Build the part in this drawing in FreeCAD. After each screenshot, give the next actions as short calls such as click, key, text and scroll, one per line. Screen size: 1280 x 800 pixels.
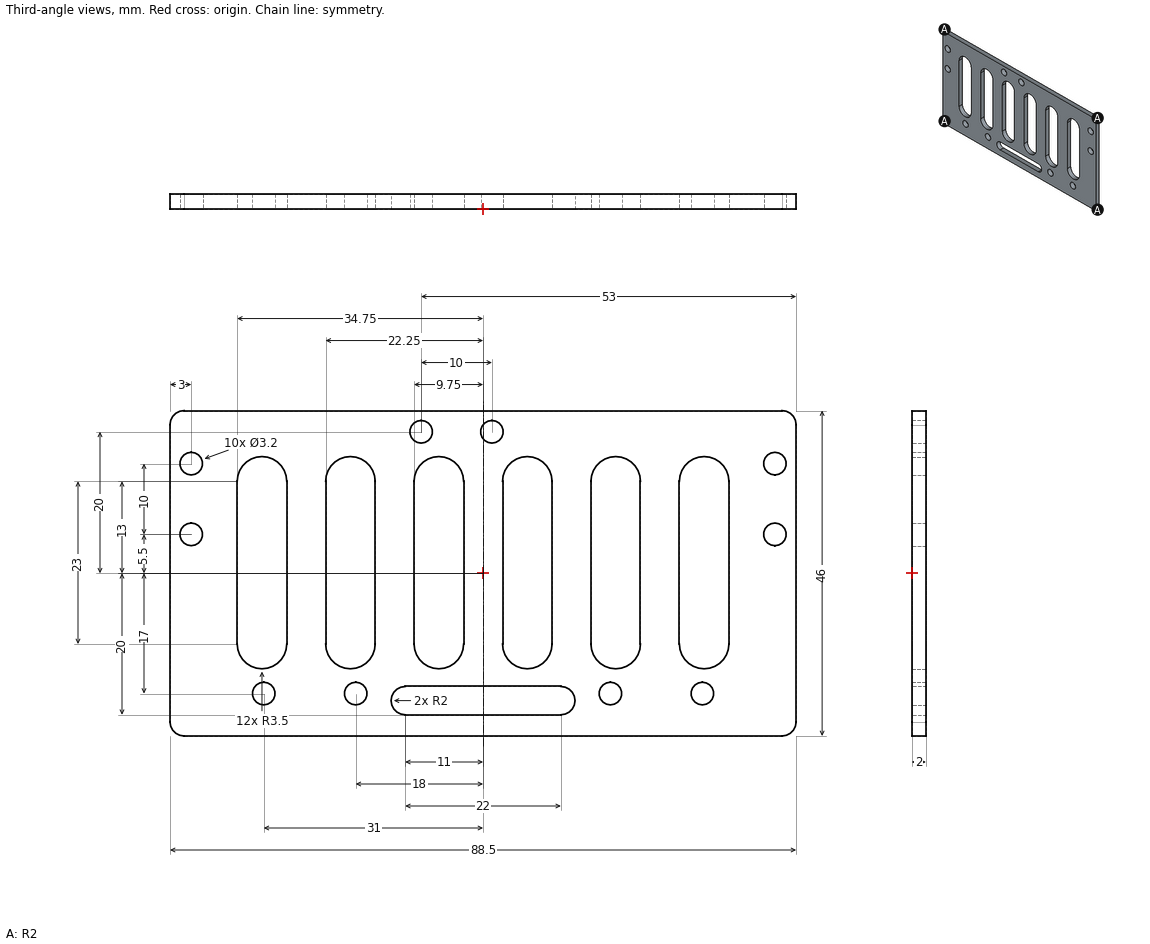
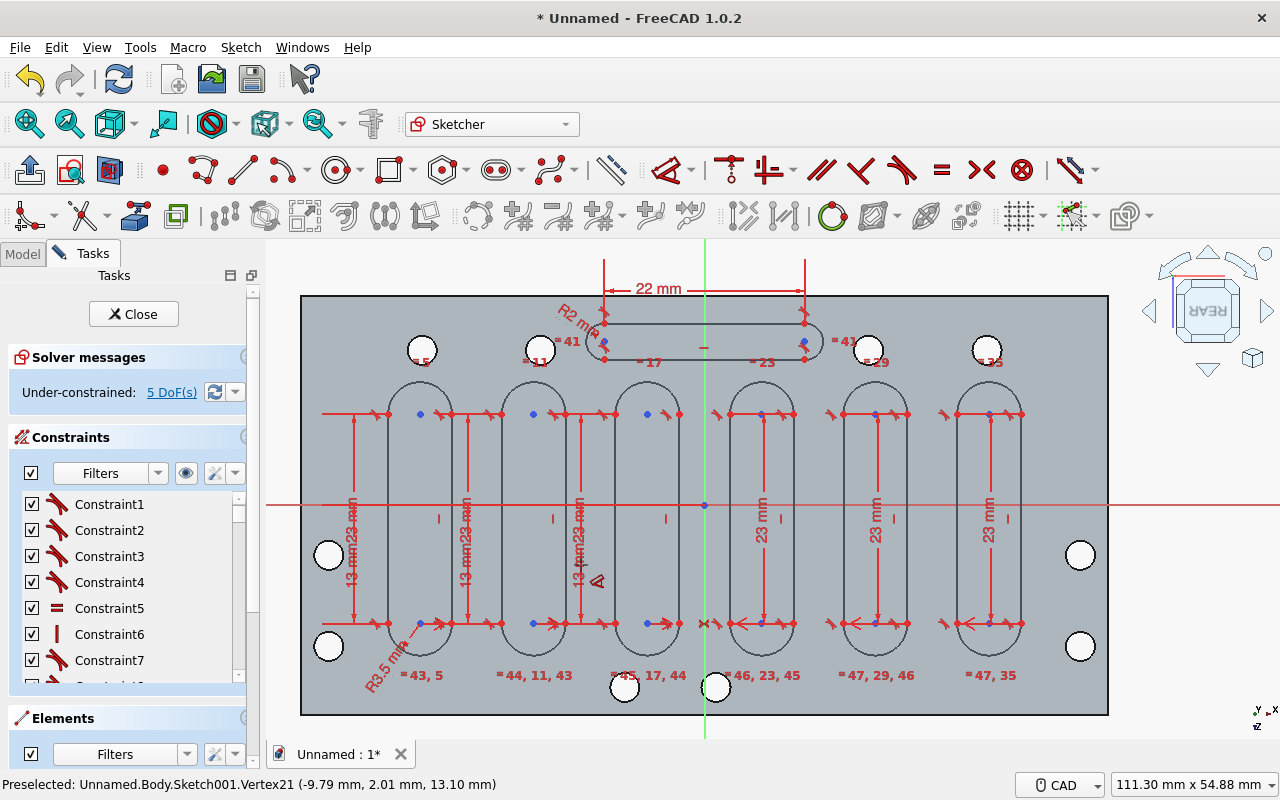
click(604, 324)
click(655, 539)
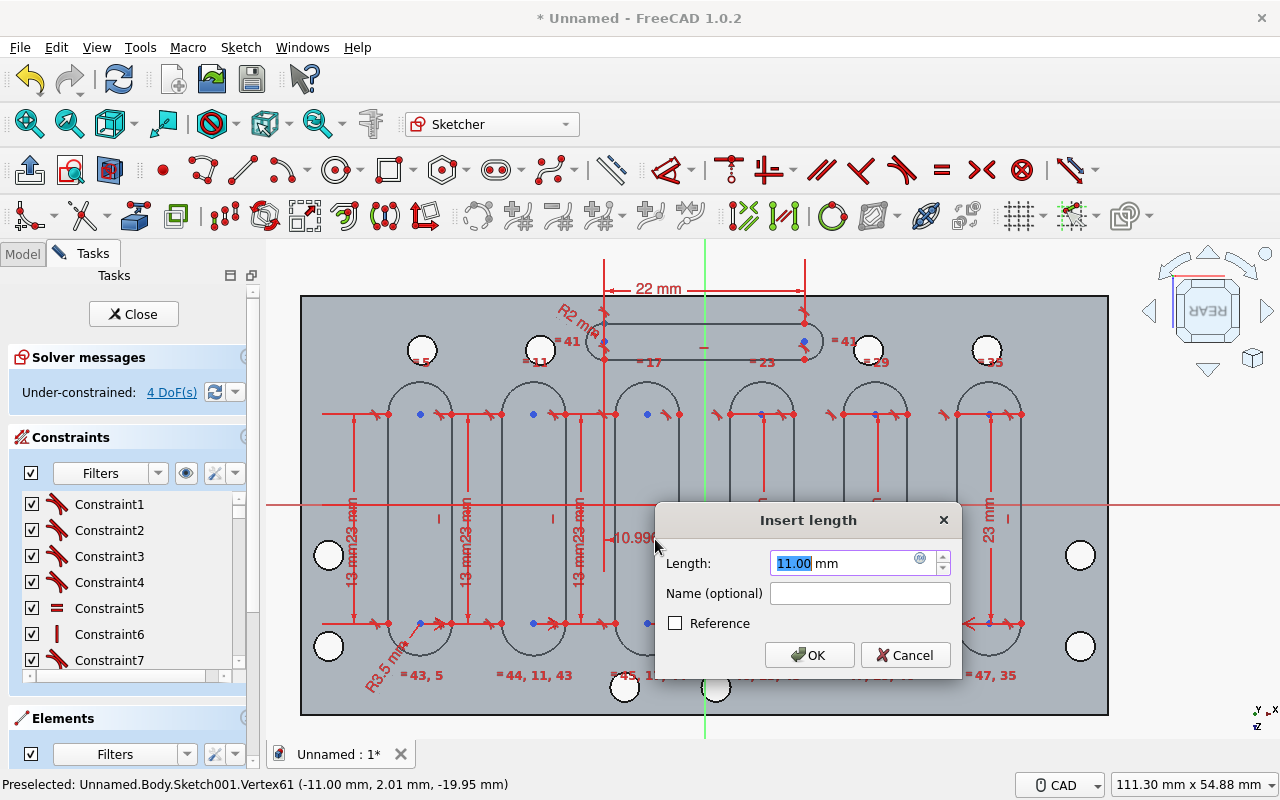
text(11)
key(Return)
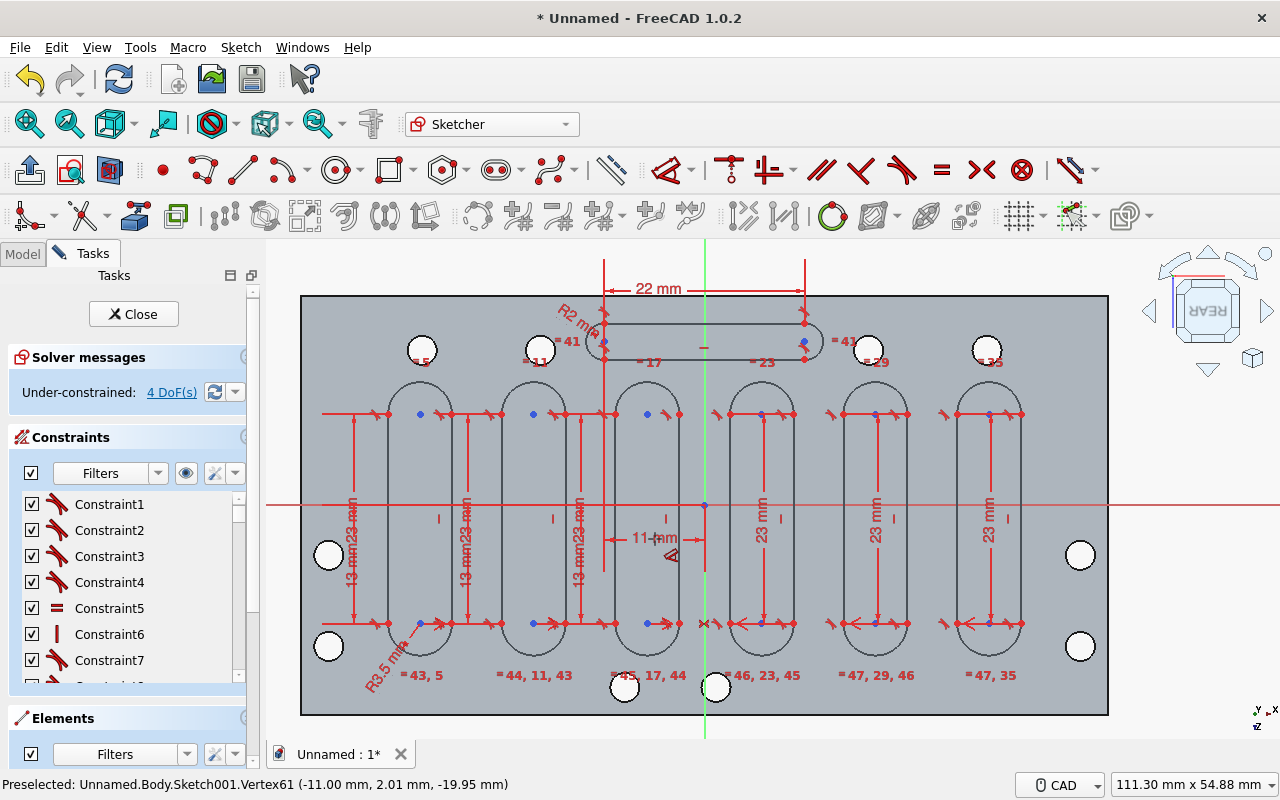
click(604, 324)
click(570, 373)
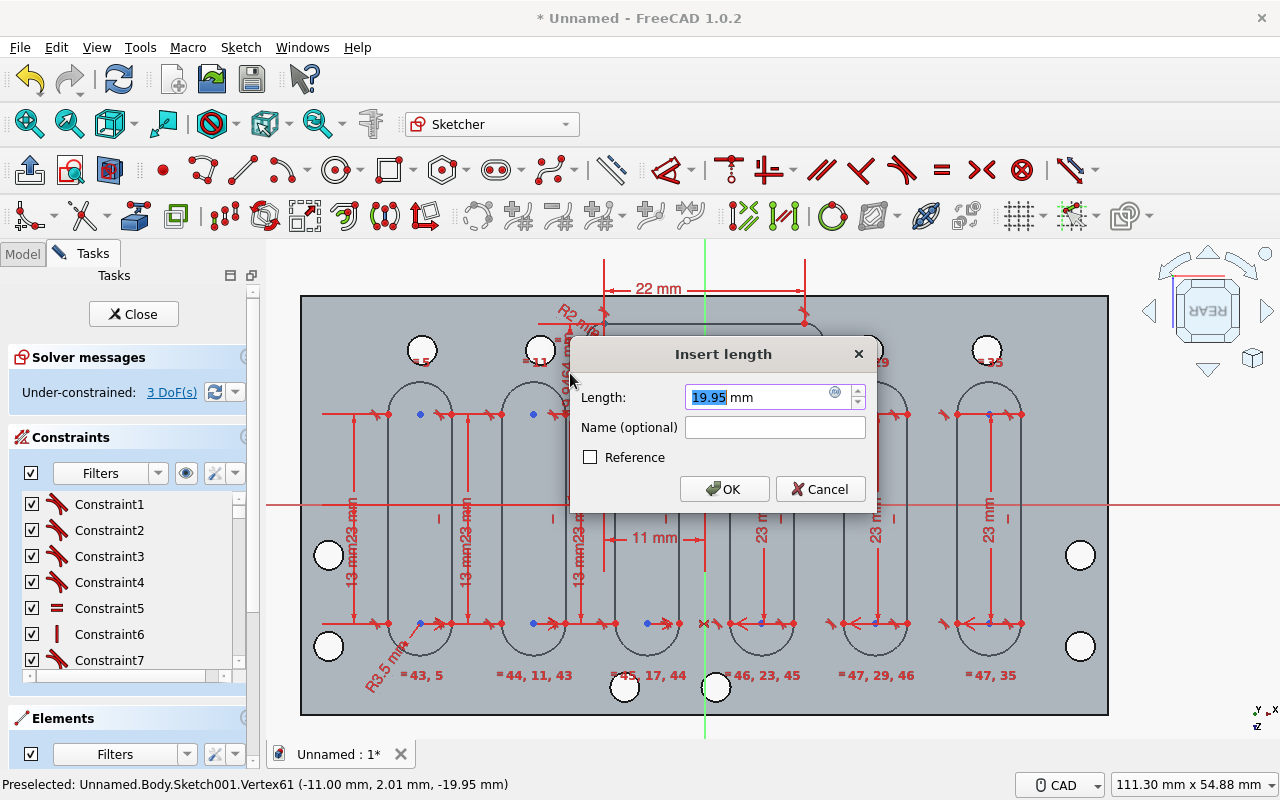
text(20)
key(Return)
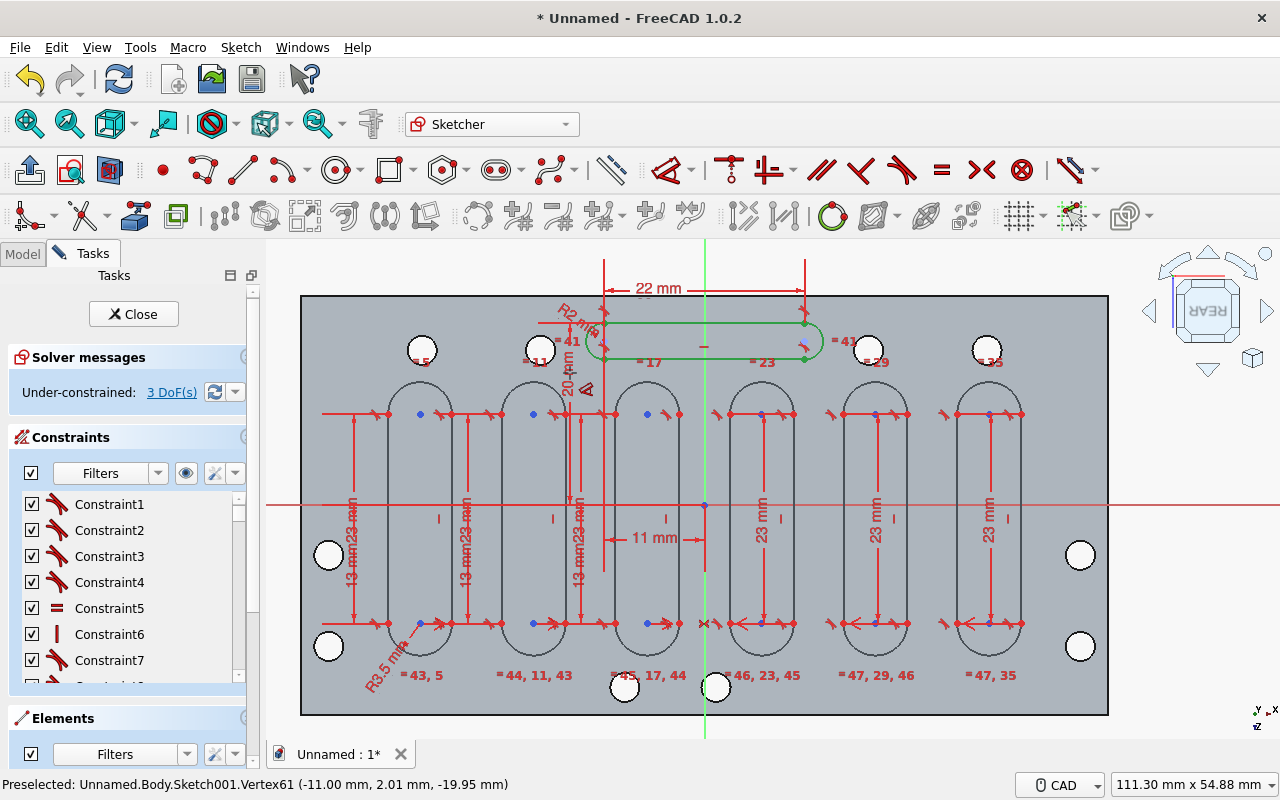
click(615, 624)
click(681, 658)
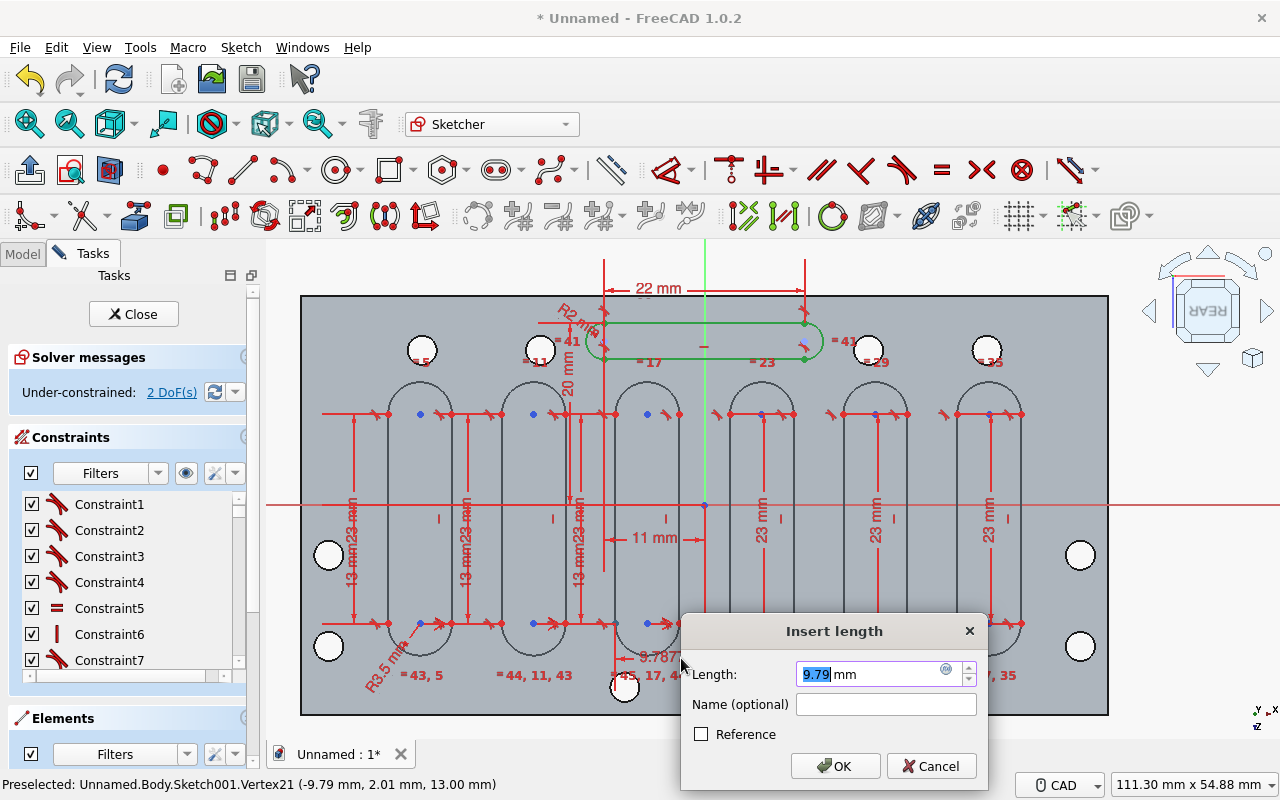
text(9.75)
key(Return)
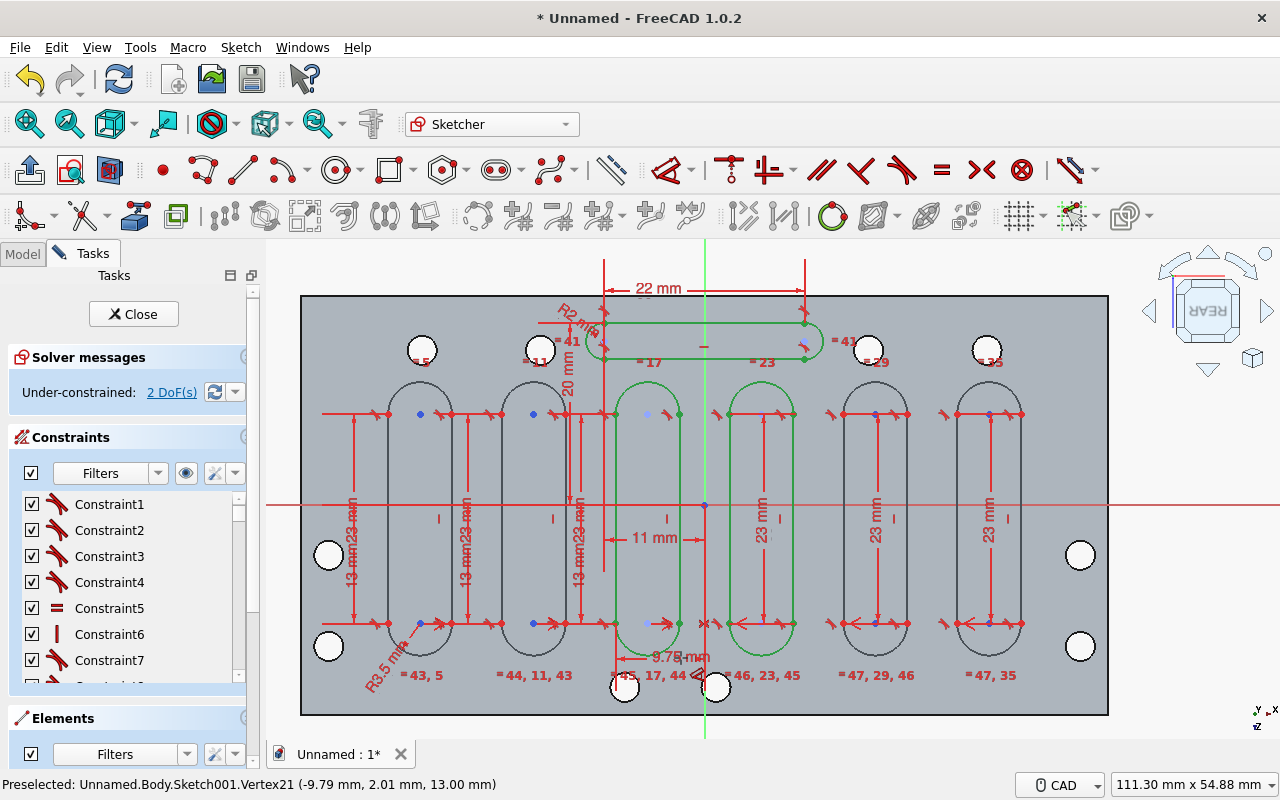
click(388, 624)
click(474, 658)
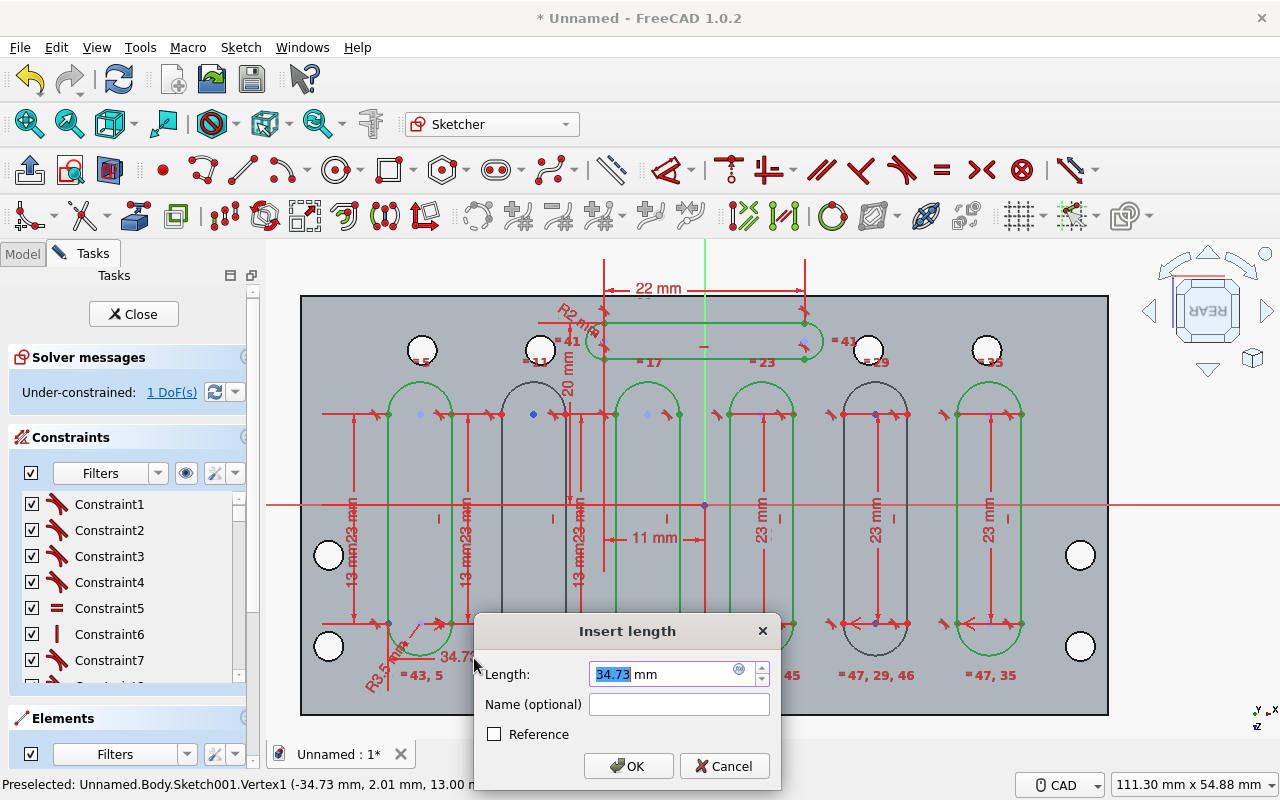
text(34.75)
key(Return)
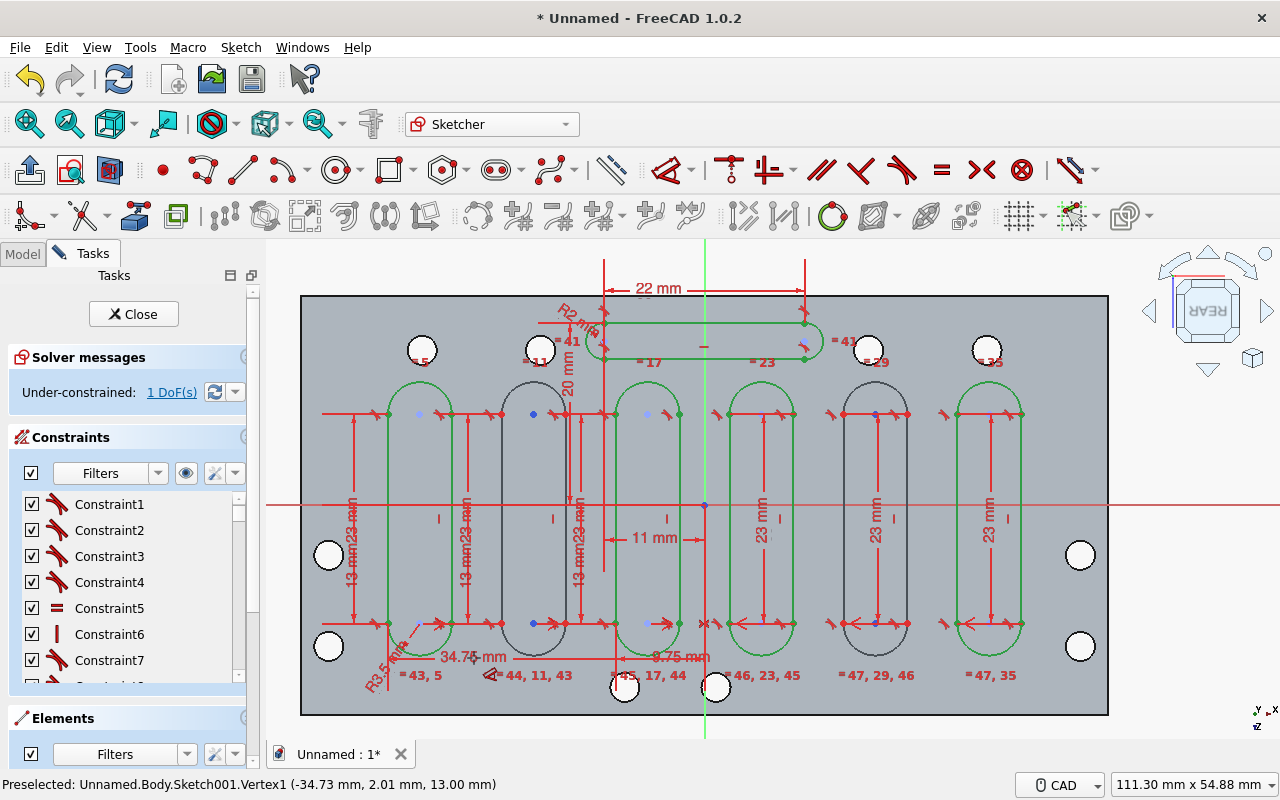
click(502, 624)
click(603, 658)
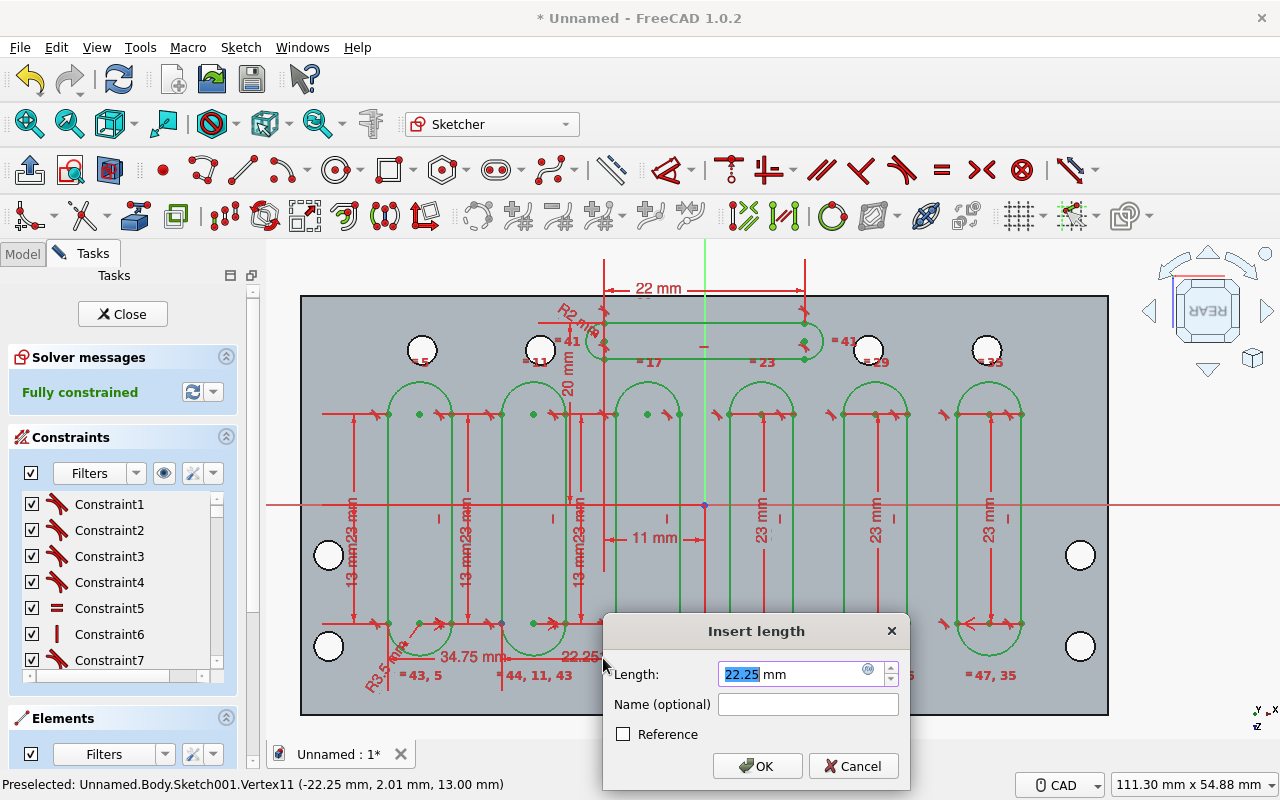
text(22.25)
key(Return)
key(Escape)